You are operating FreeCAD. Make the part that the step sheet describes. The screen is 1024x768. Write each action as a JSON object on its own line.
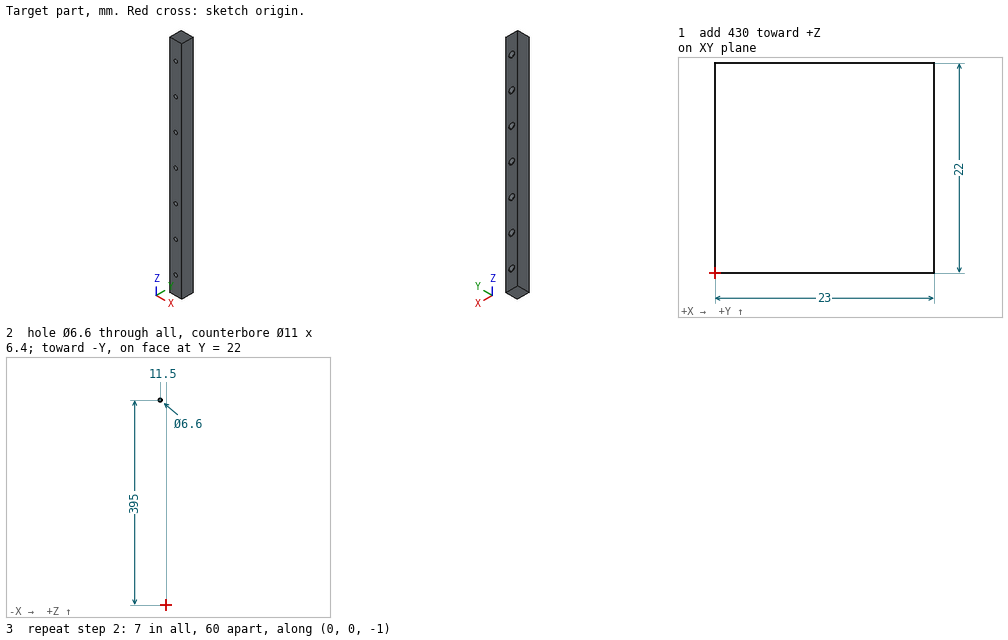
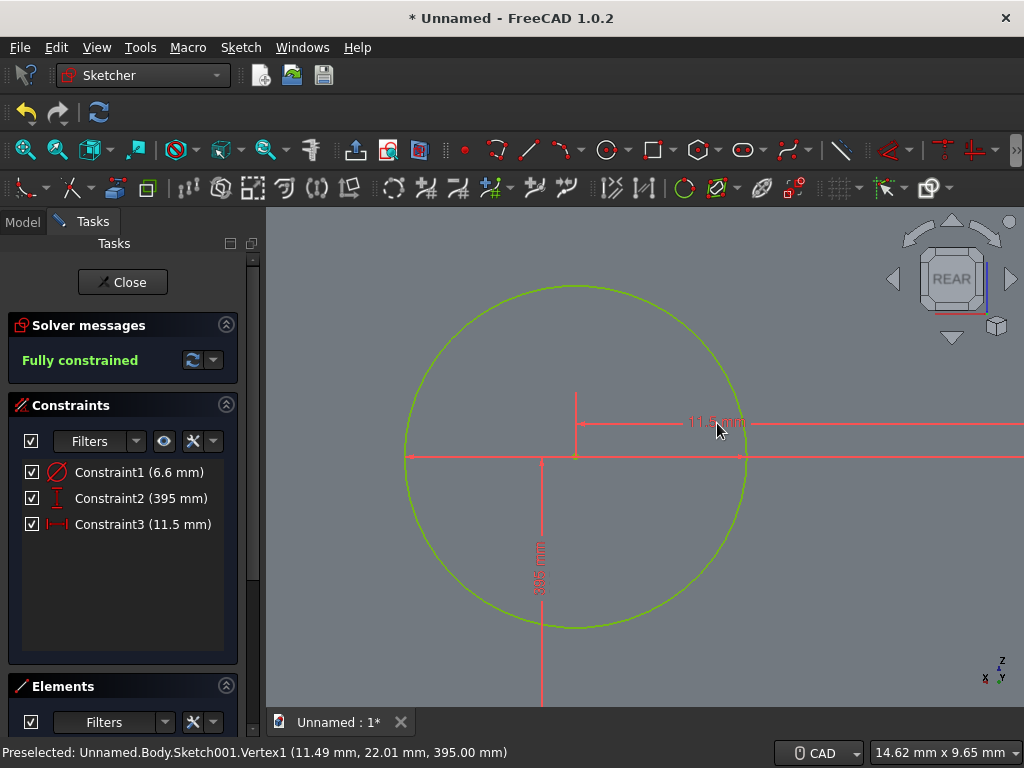
{"action": "left_click", "coordinate": [123, 282]}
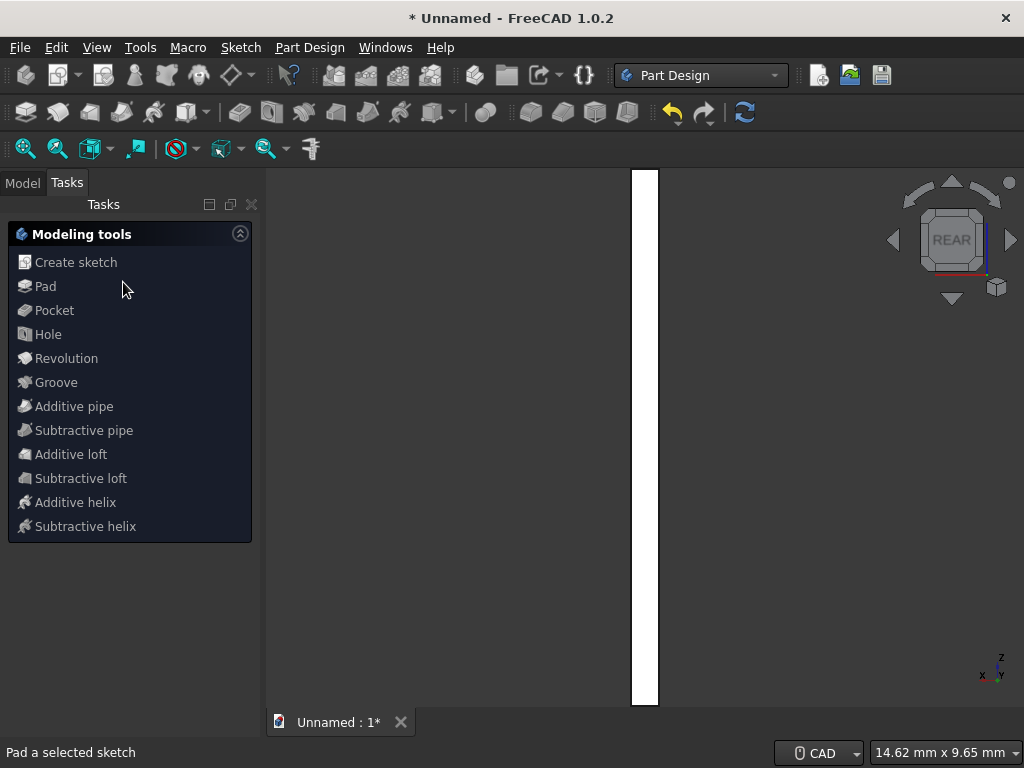
{"action": "left_click", "coordinate": [272, 112]}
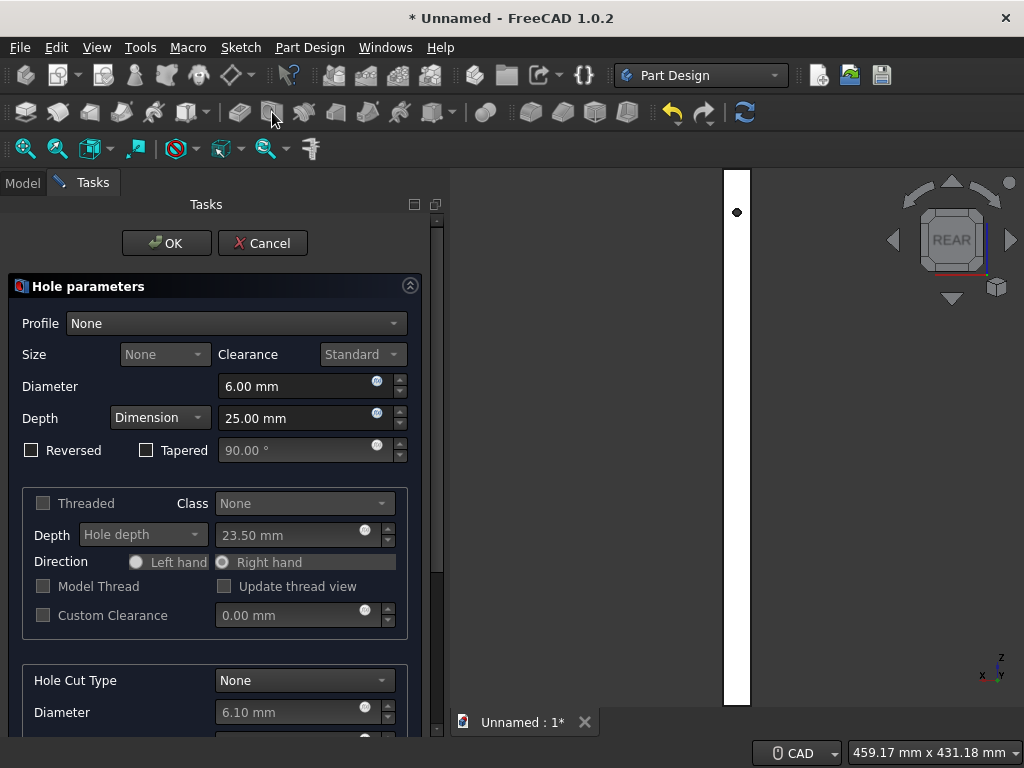
{"action": "triple_click", "coordinate": [305, 386]}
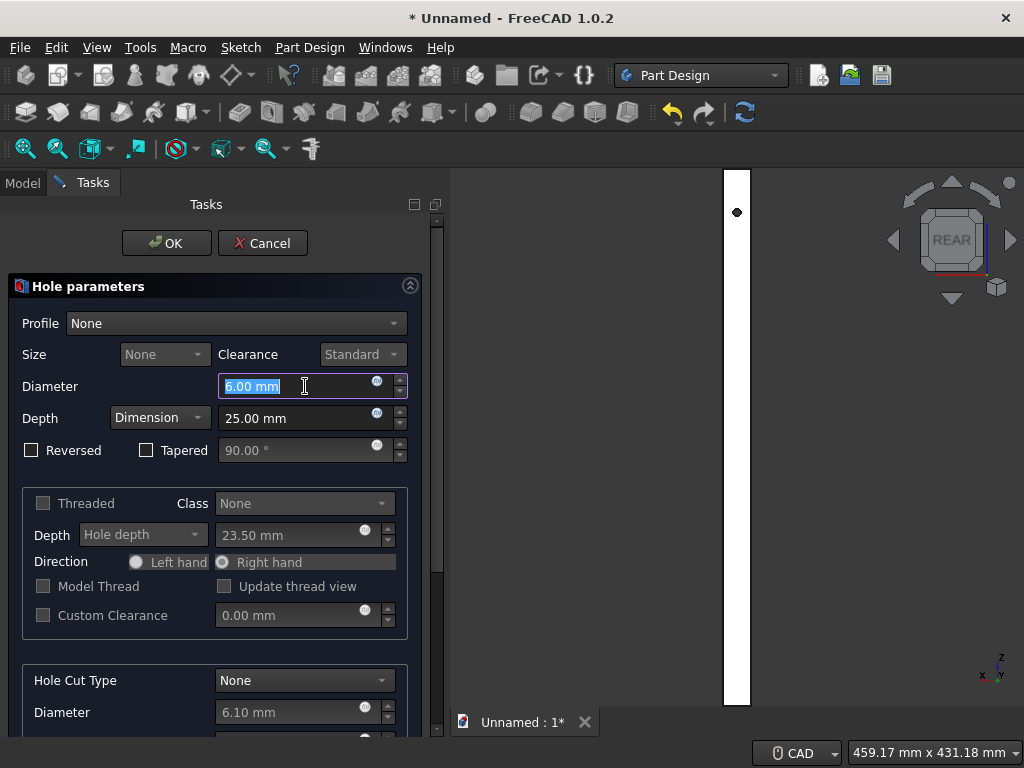
{"action": "type", "text": "6.6"}
{"action": "key", "text": "Tab"}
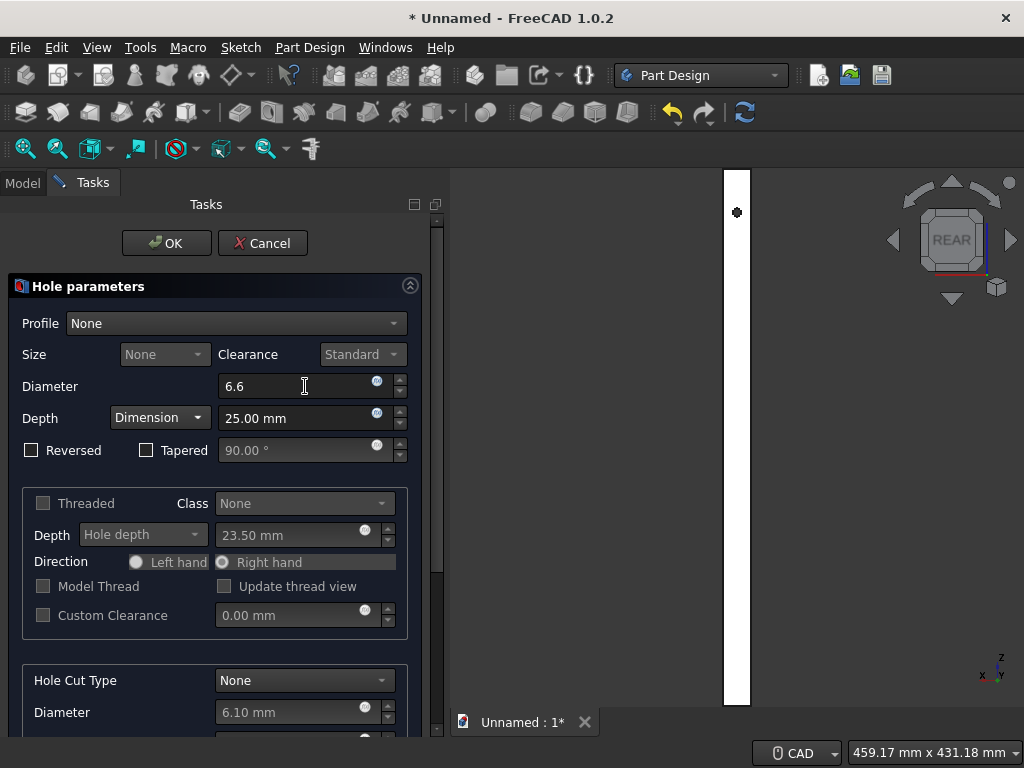
{"action": "left_click", "coordinate": [161, 418]}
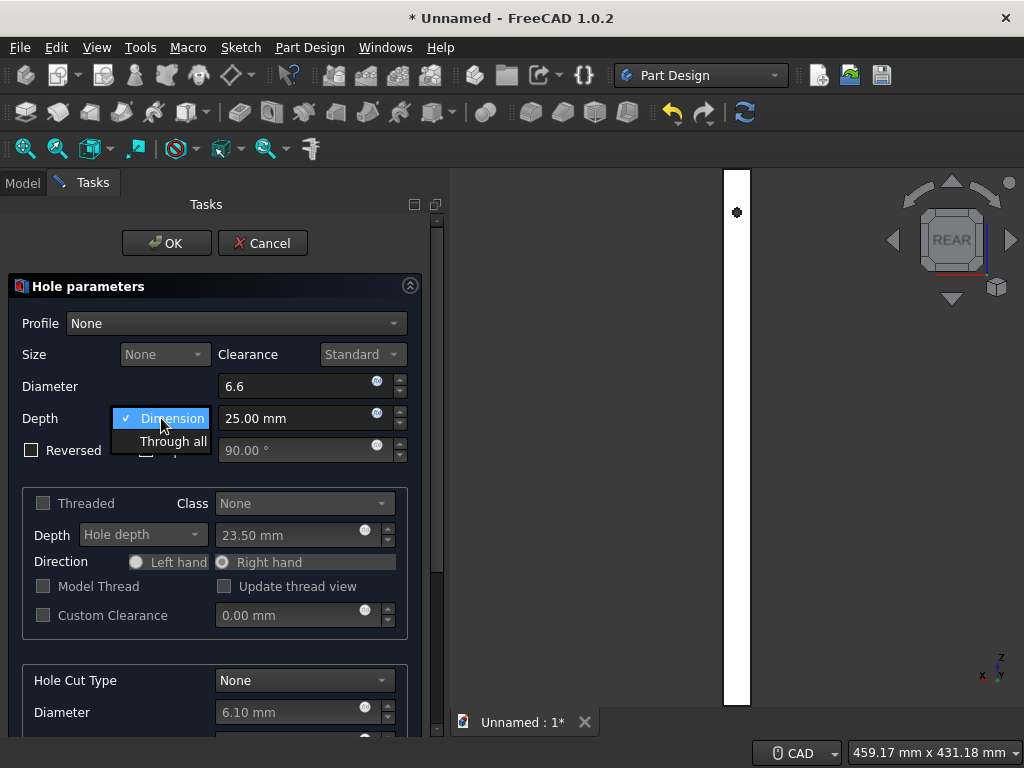
{"action": "left_click", "coordinate": [160, 442]}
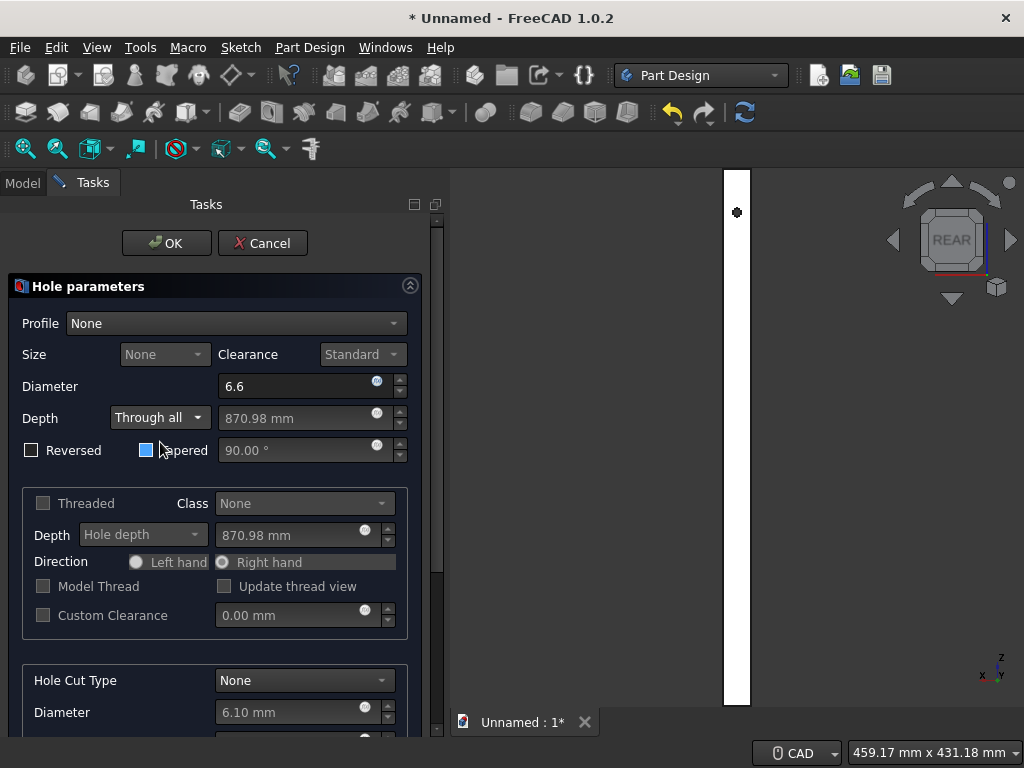
{"action": "left_click", "coordinate": [306, 680]}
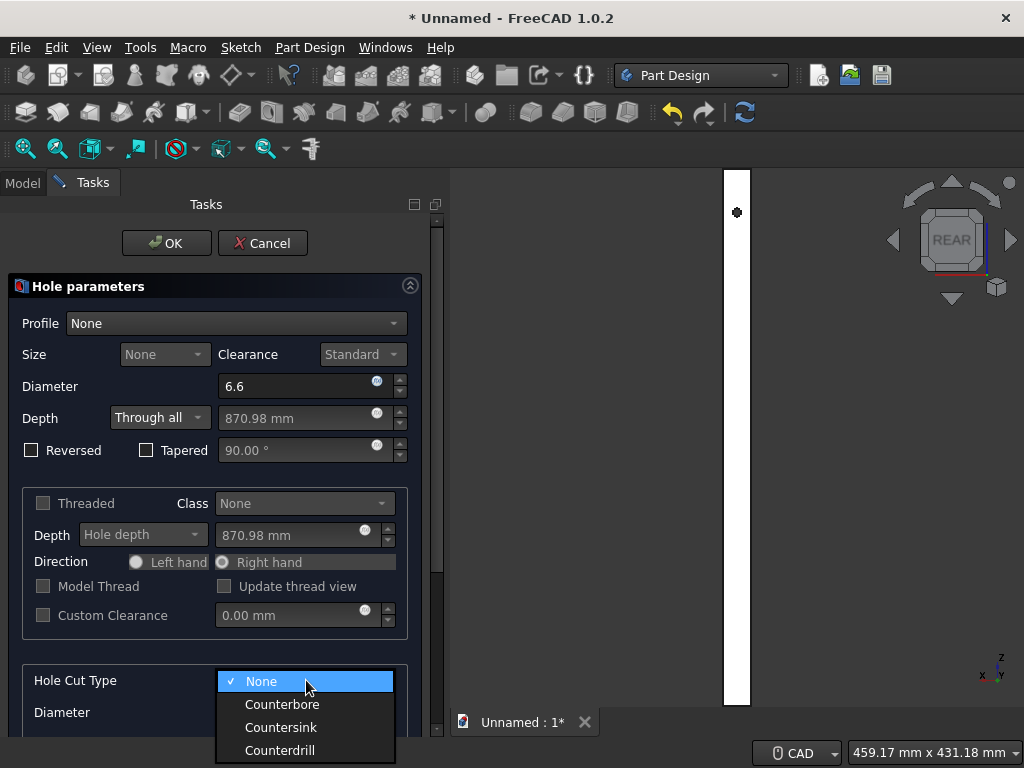
{"action": "left_click", "coordinate": [304, 704]}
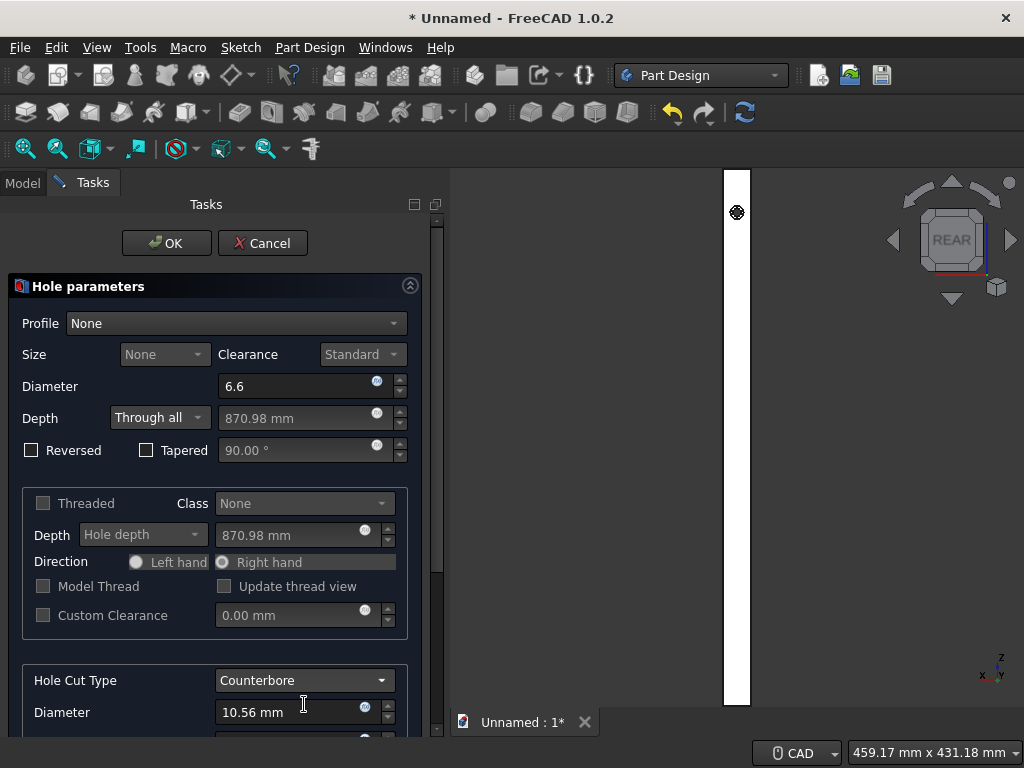
{"action": "triple_click", "coordinate": [298, 712]}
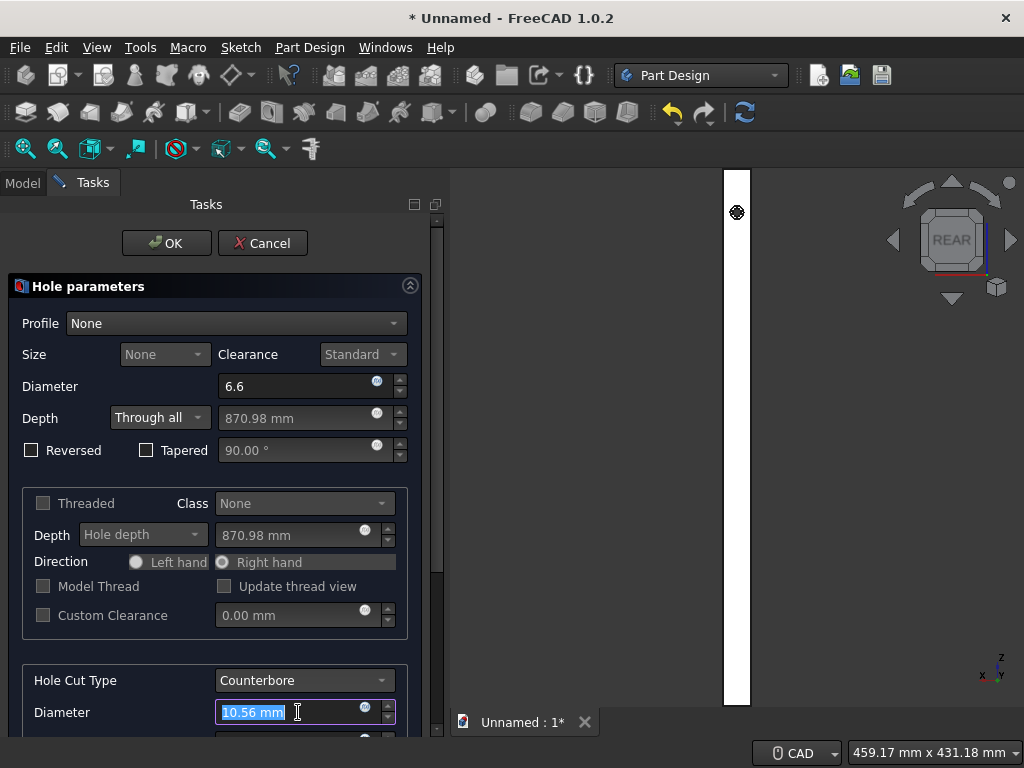
{"action": "type", "text": "11"}
{"action": "key", "text": "Tab"}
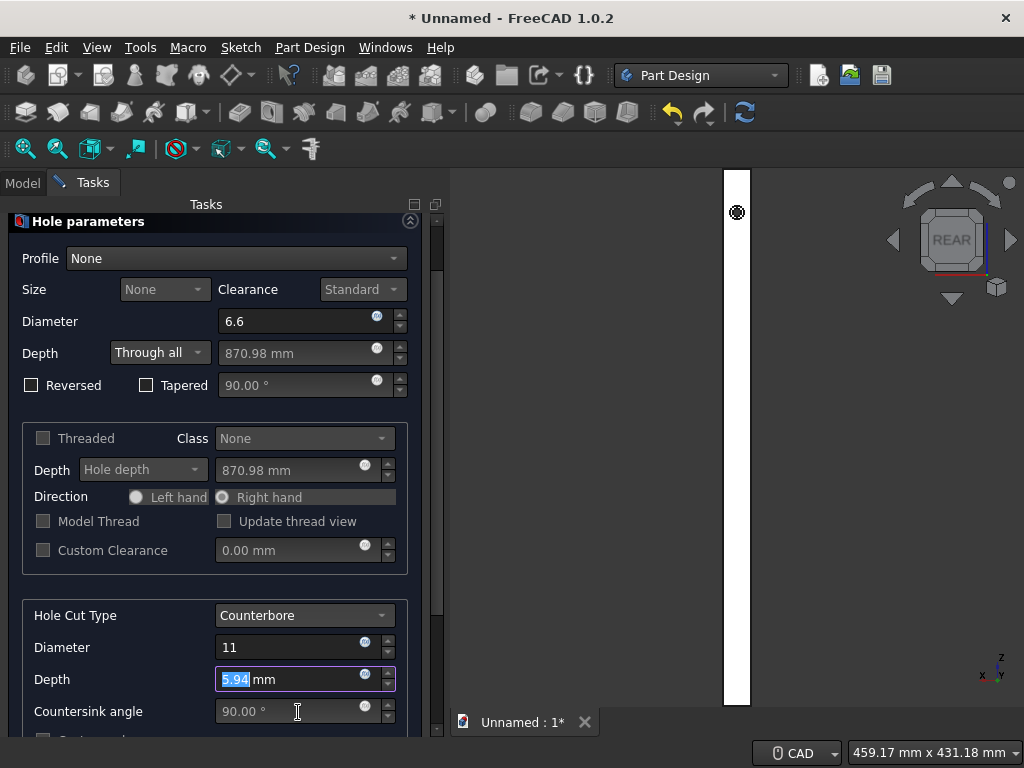
{"action": "type", "text": "6.4"}
{"action": "key", "text": "Tab"}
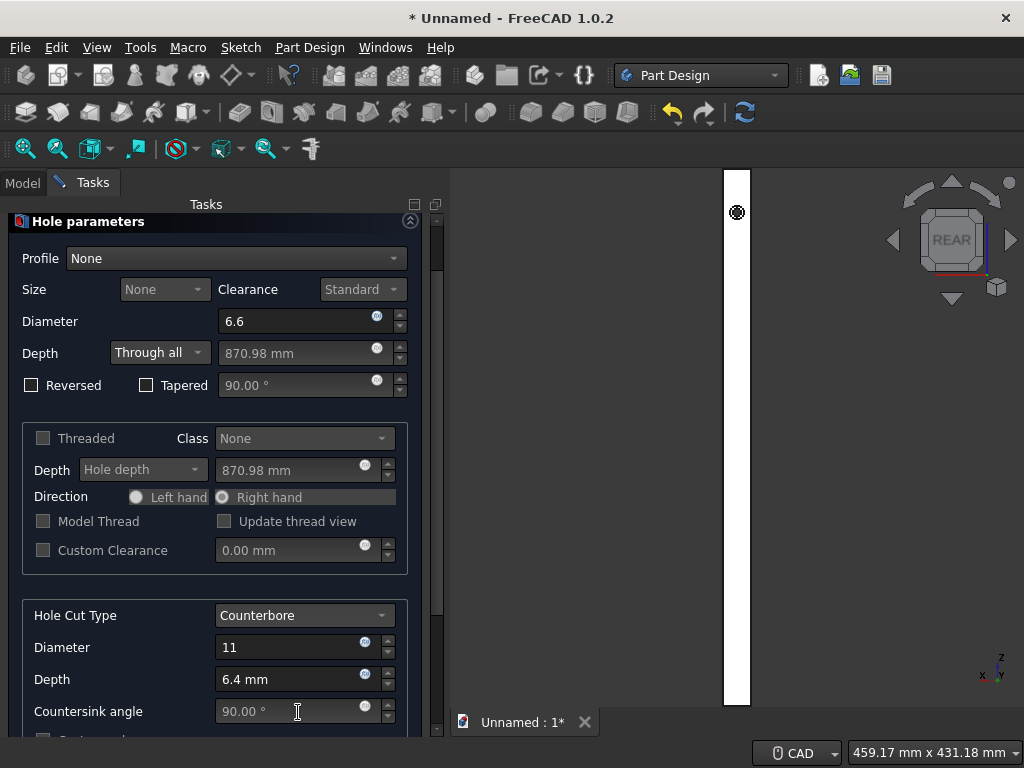
{"action": "scroll", "coordinate": [437, 475], "scroll_direction": "up", "scroll_amount": 2}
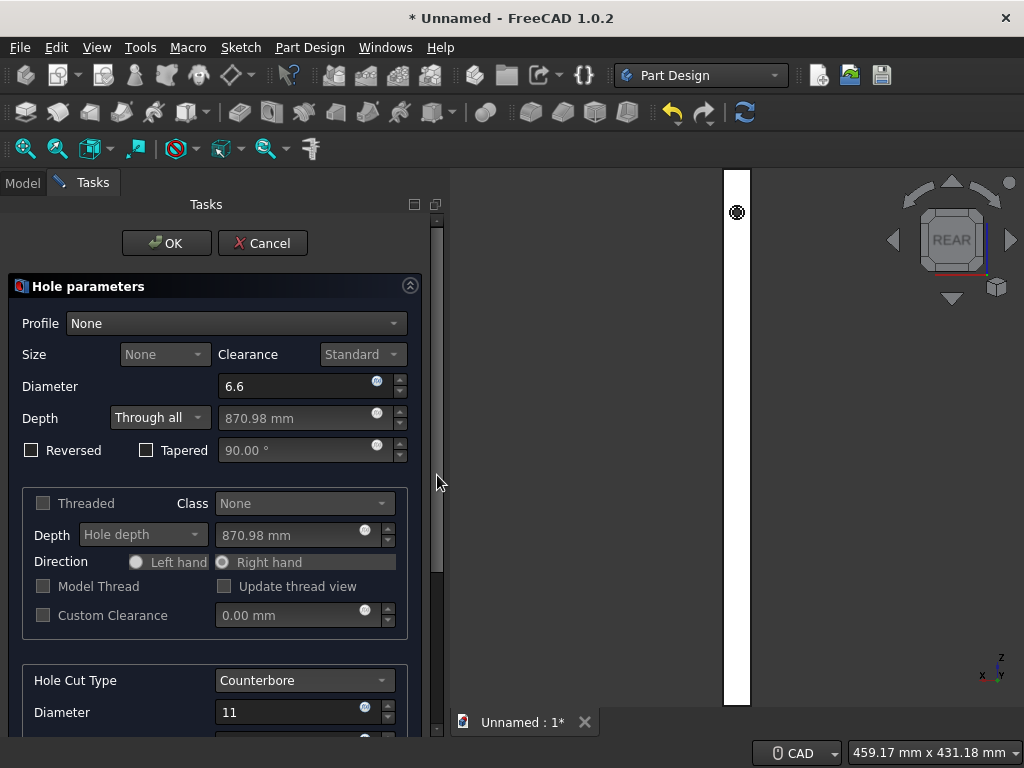
{"action": "left_click", "coordinate": [167, 243]}